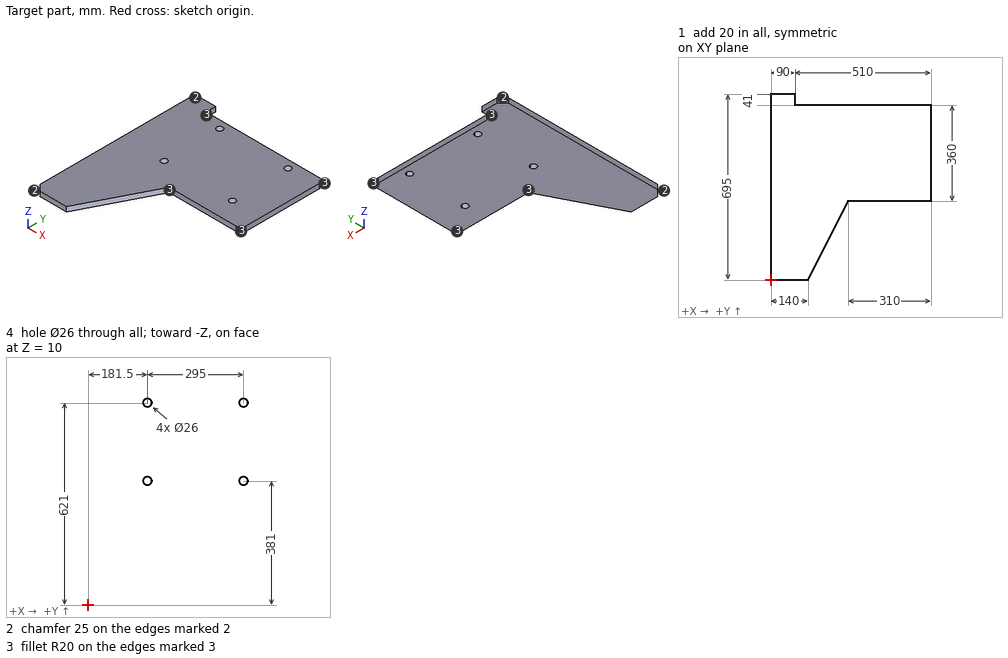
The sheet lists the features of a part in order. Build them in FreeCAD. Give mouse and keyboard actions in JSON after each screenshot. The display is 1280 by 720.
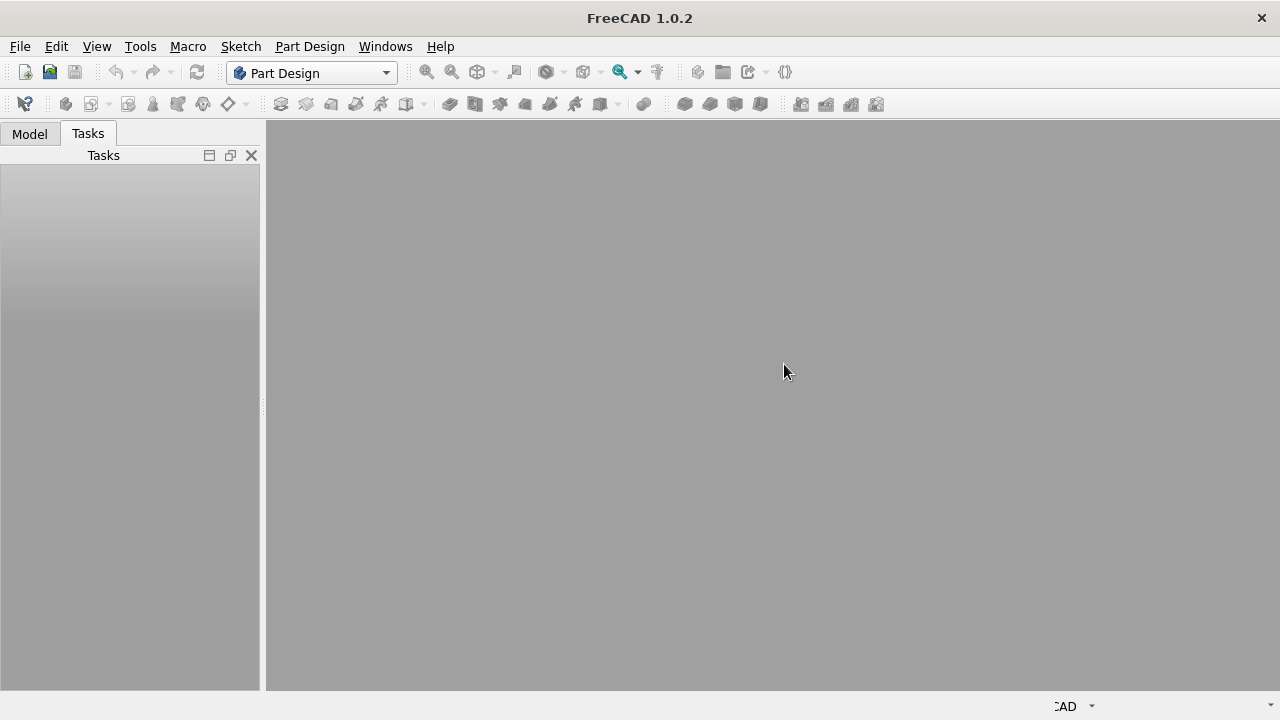
{"action": "left_click", "coordinate": [25, 72]}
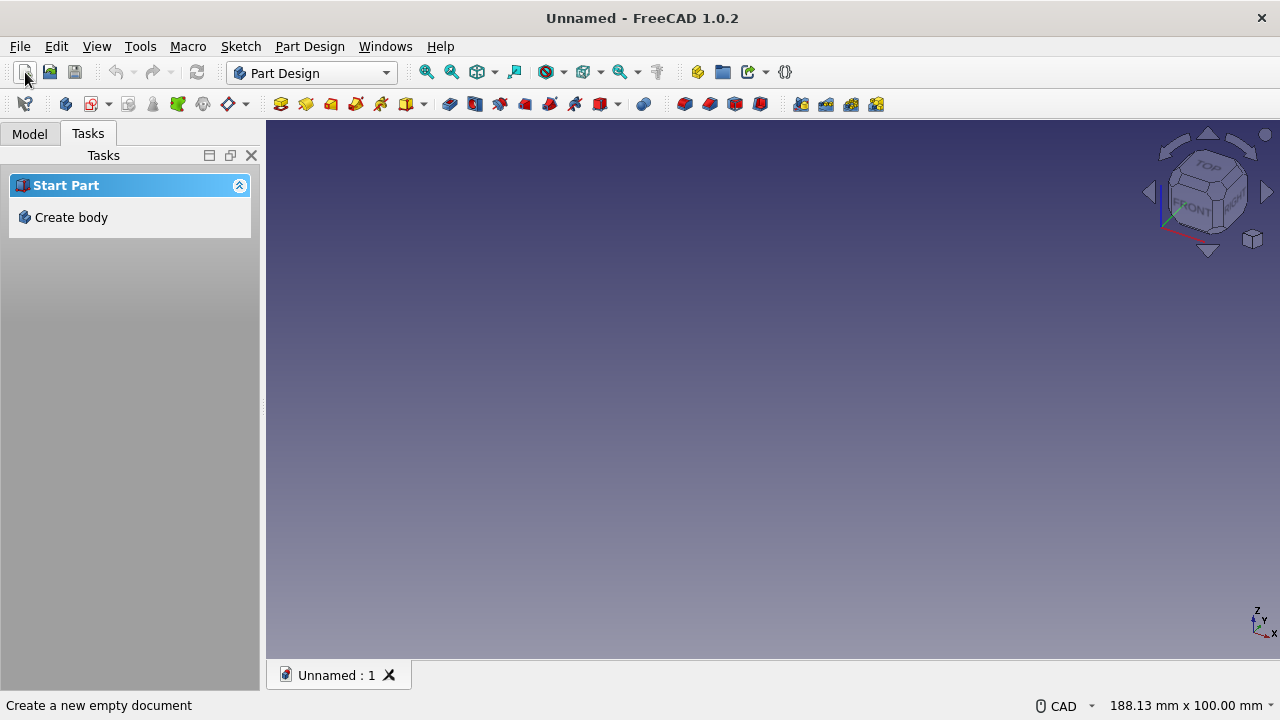
{"action": "left_click", "coordinate": [90, 104]}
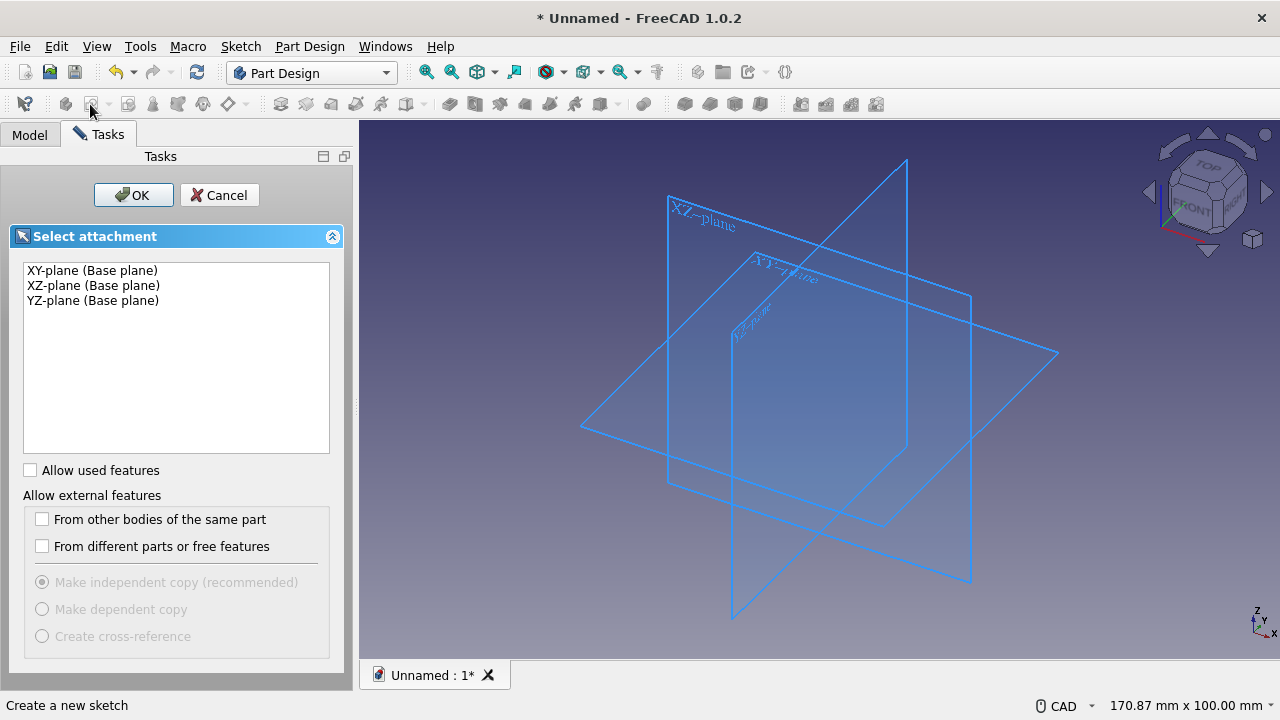
{"action": "left_click", "coordinate": [84, 270]}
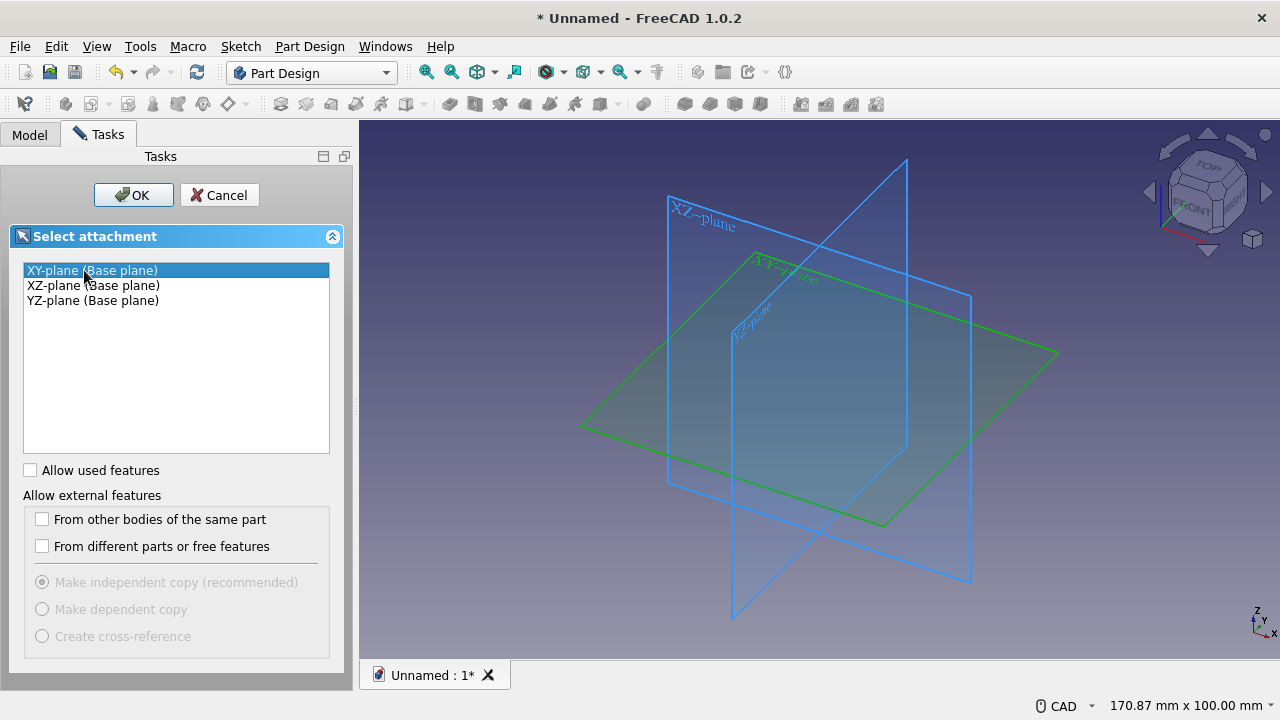
{"action": "left_click", "coordinate": [134, 195]}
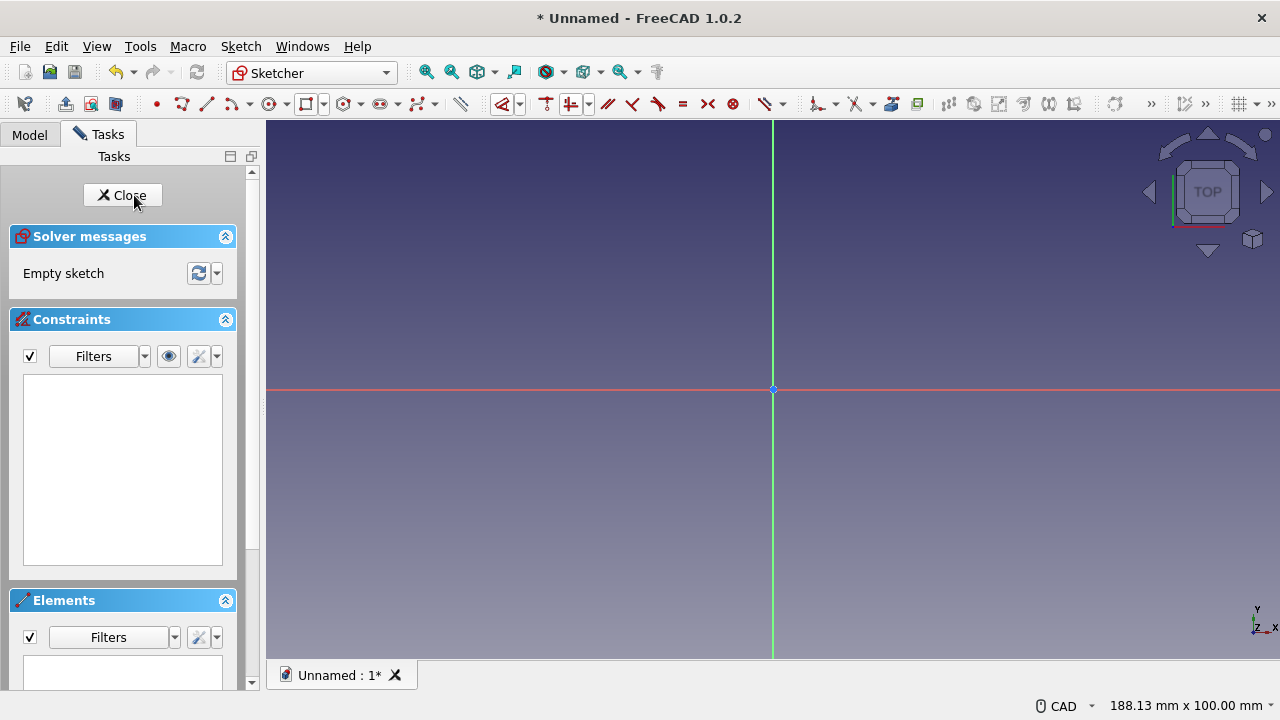
{"action": "scroll", "coordinate": [536, 576], "scroll_direction": "down", "scroll_amount": 12}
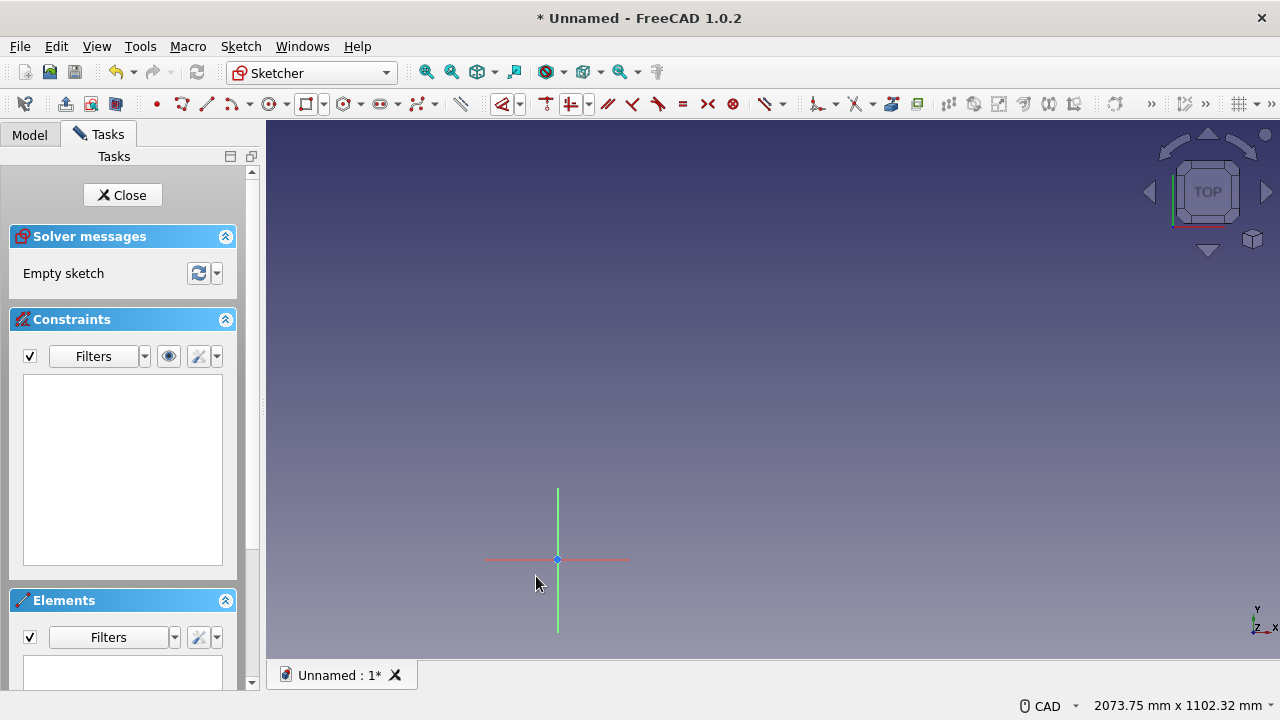
{"action": "left_click", "coordinate": [182, 104]}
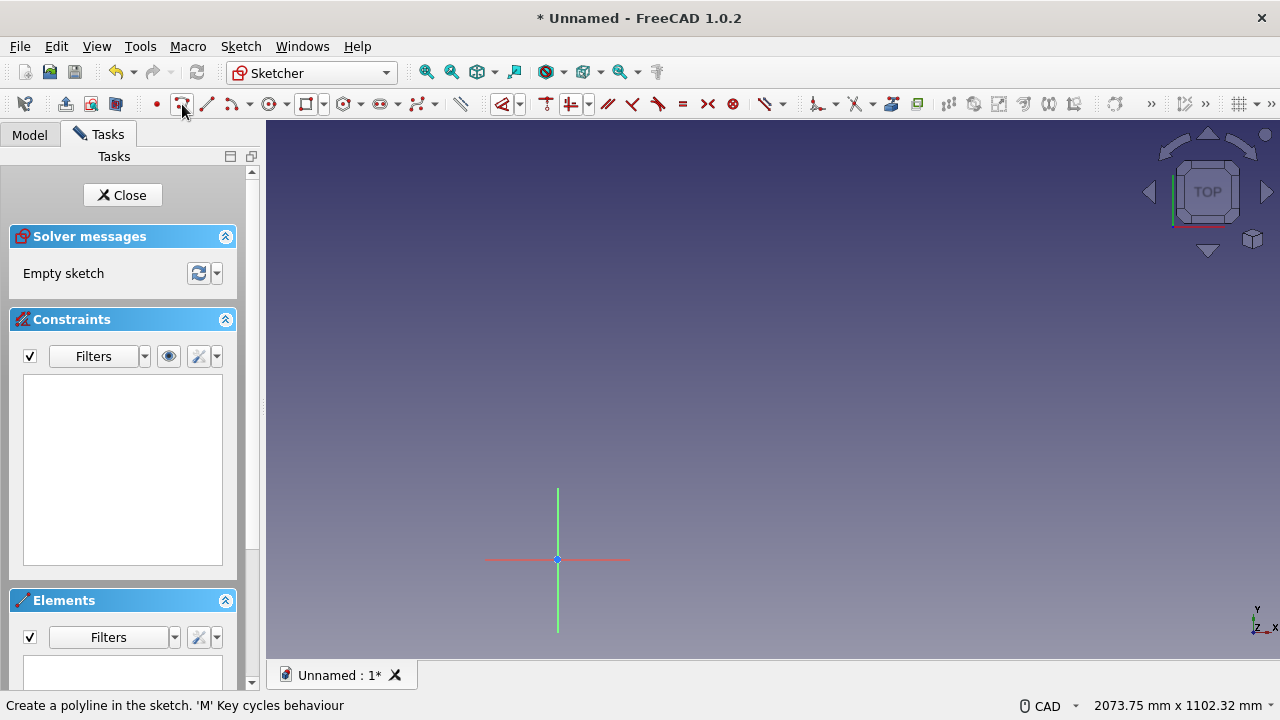
{"action": "left_click", "coordinate": [558, 560]}
{"action": "left_click", "coordinate": [626, 551]}
{"action": "left_click", "coordinate": [700, 416]}
{"action": "left_click", "coordinate": [851, 416]}
{"action": "left_click", "coordinate": [851, 240]}
{"action": "left_click", "coordinate": [602, 240]}
{"action": "left_click", "coordinate": [602, 220]}
{"action": "left_click", "coordinate": [567, 220]}
{"action": "left_click", "coordinate": [558, 560]}
{"action": "key", "text": "Escape"}
{"action": "key", "text": "Escape"}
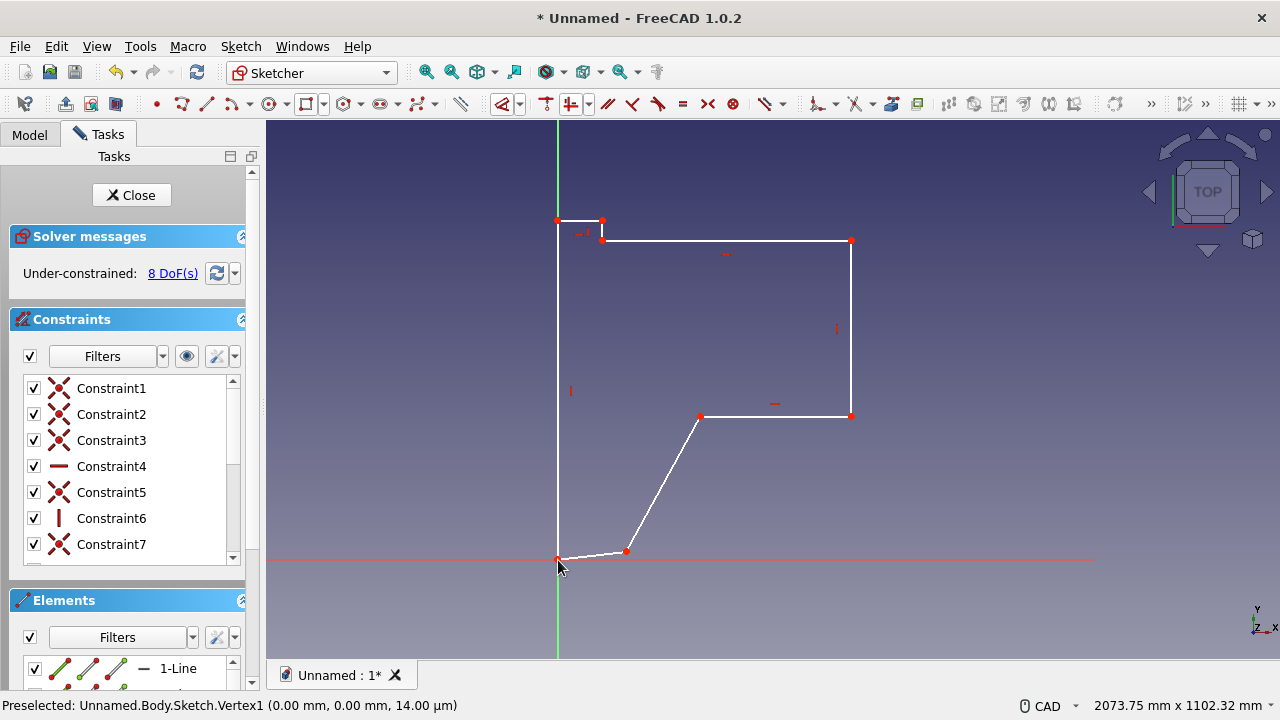
{"action": "left_click", "coordinate": [578, 557]}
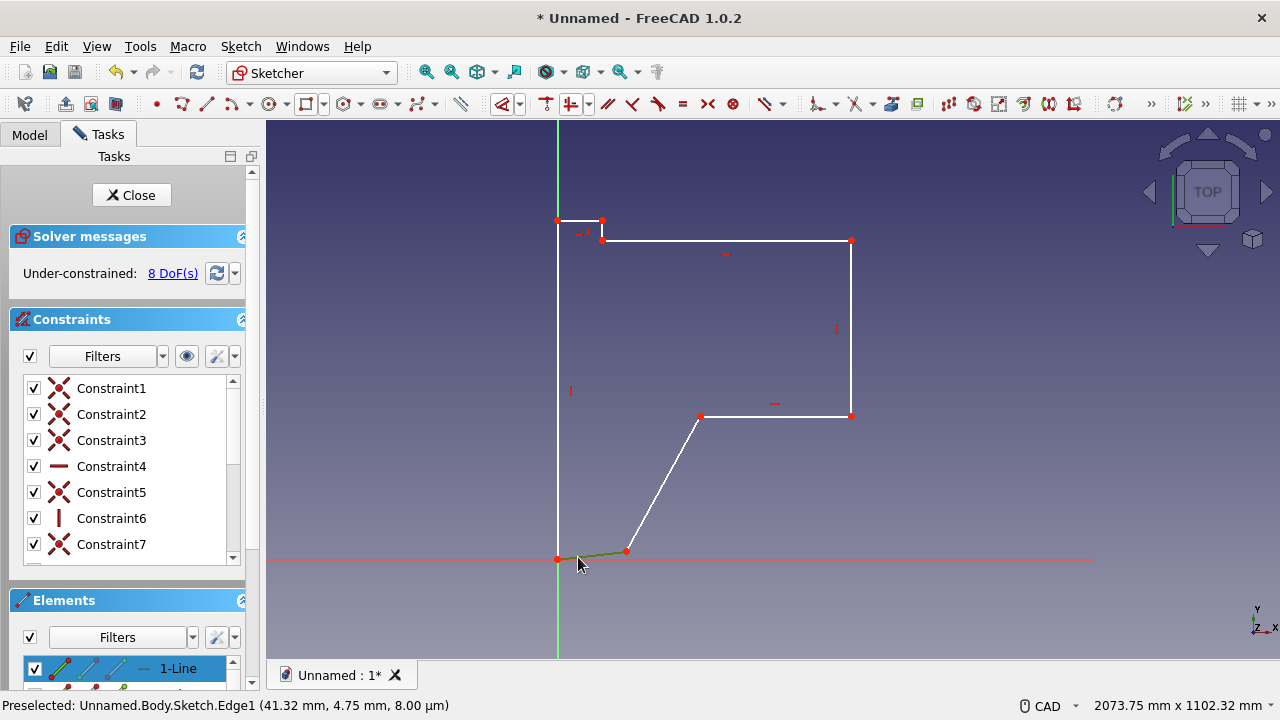
{"action": "key", "text": "h"}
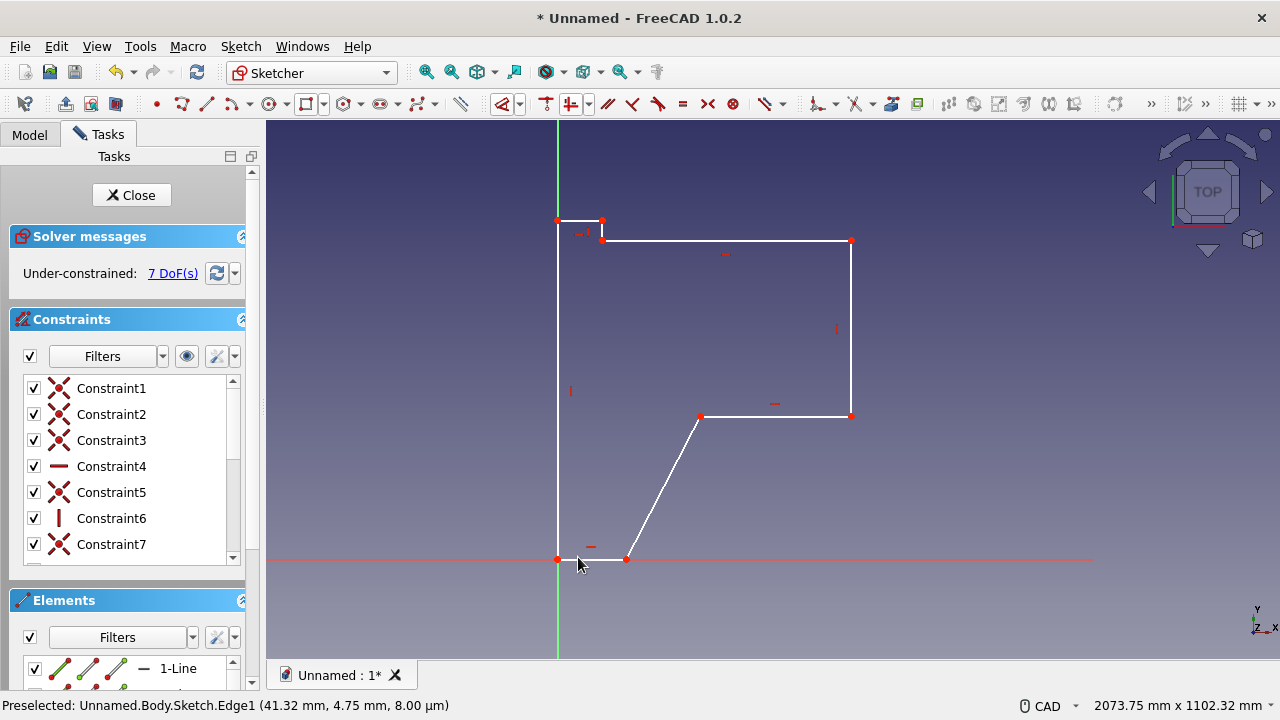
{"action": "scroll", "coordinate": [602, 231], "scroll_direction": "up", "scroll_amount": 4}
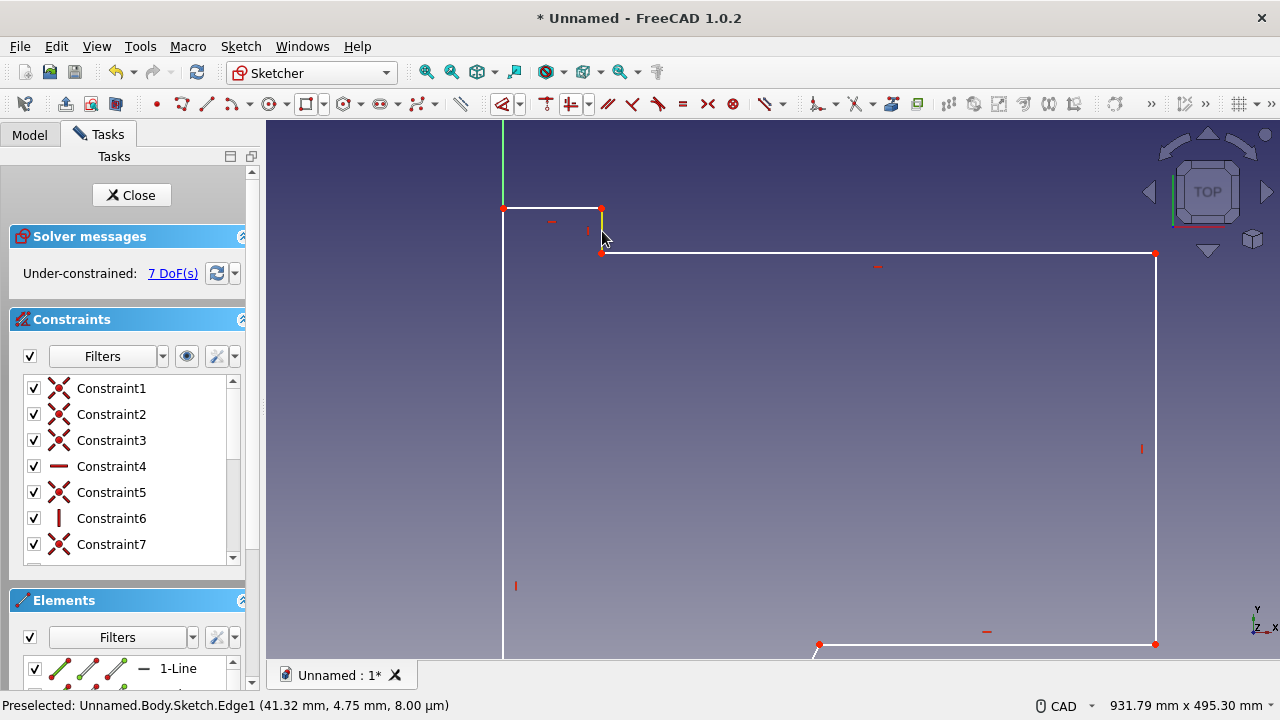
{"action": "left_click", "coordinate": [602, 231]}